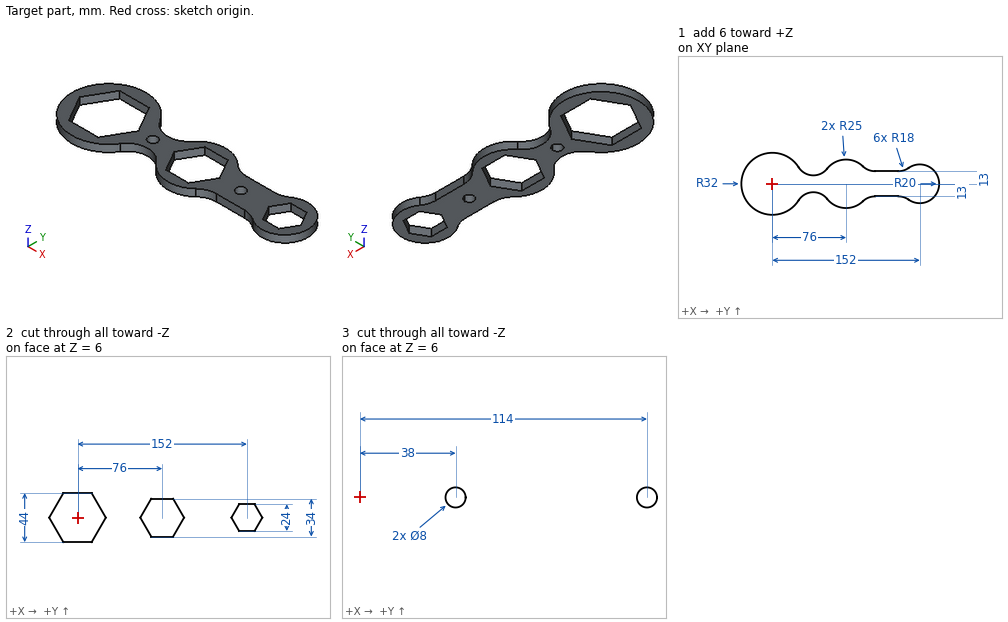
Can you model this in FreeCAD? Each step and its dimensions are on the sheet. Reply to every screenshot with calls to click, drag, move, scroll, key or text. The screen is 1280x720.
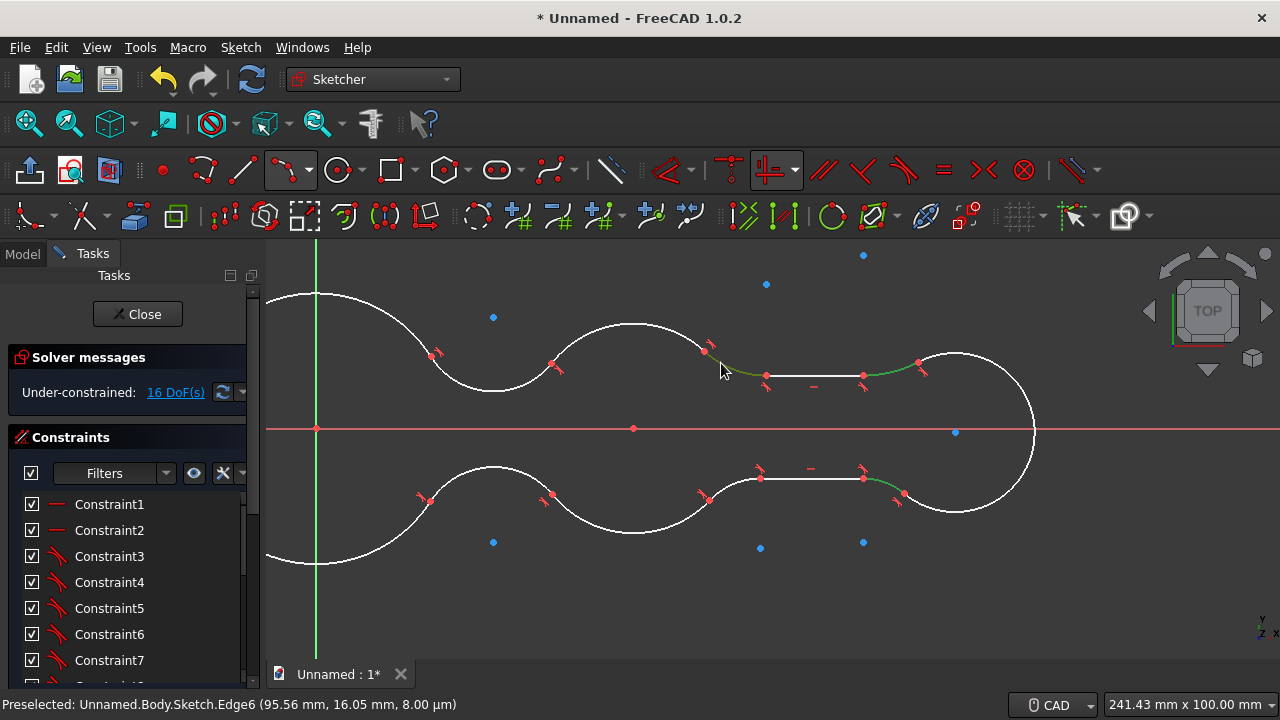
click(462, 385)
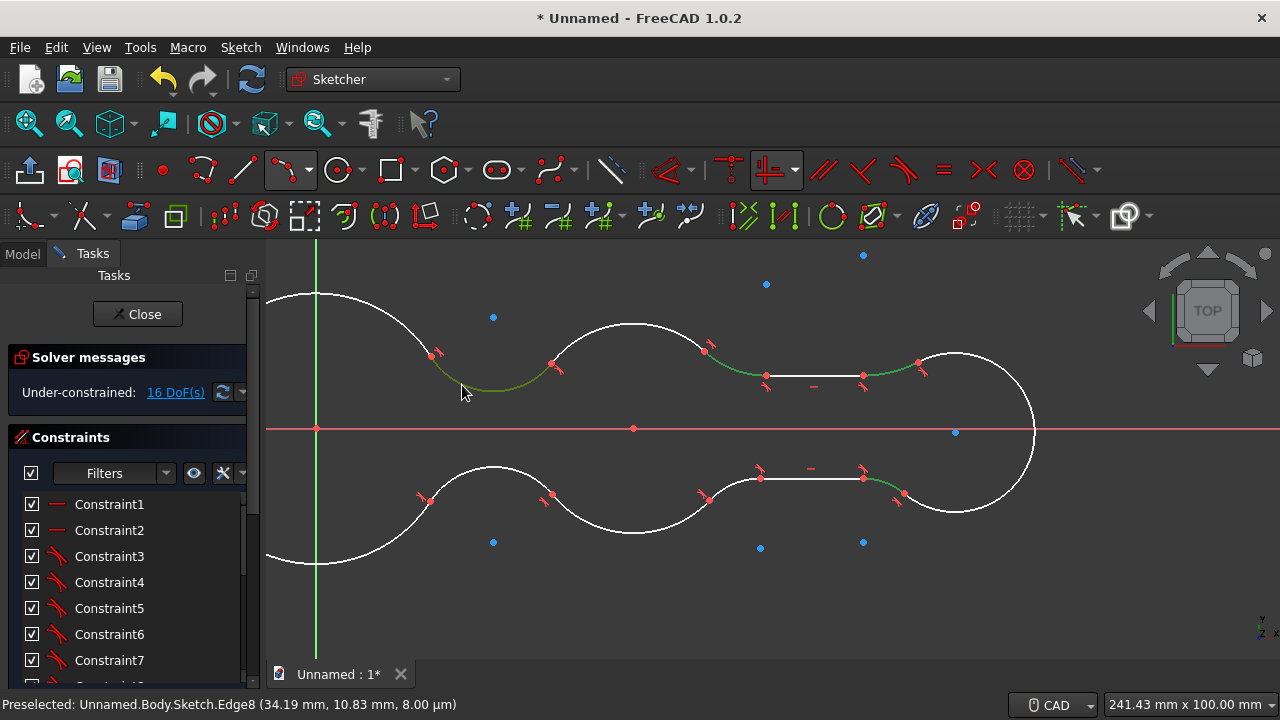
click(518, 471)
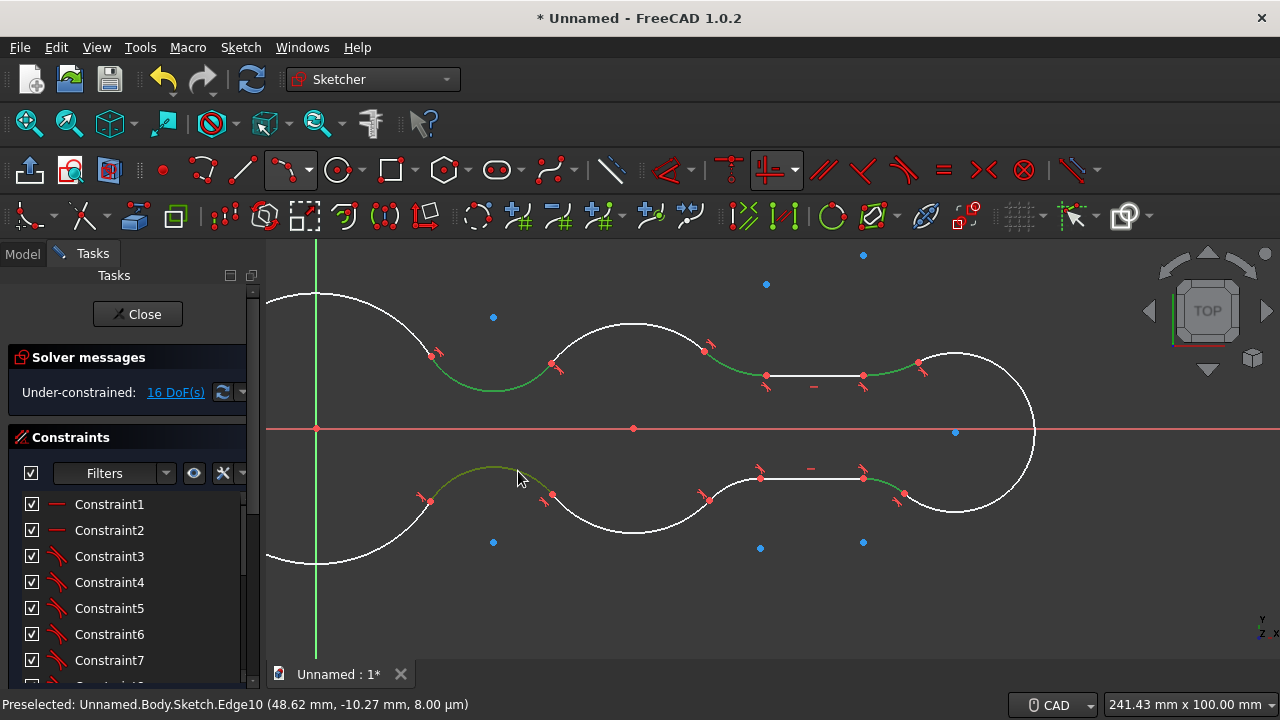
click(744, 481)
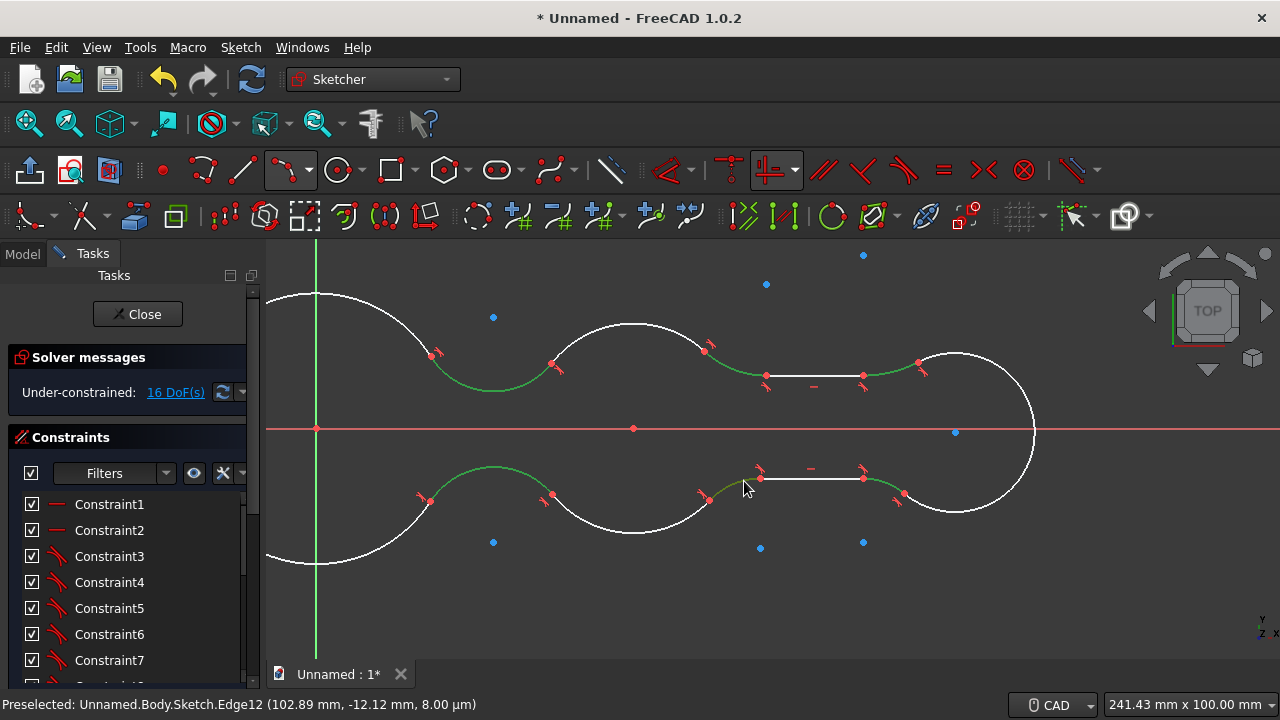
click(944, 170)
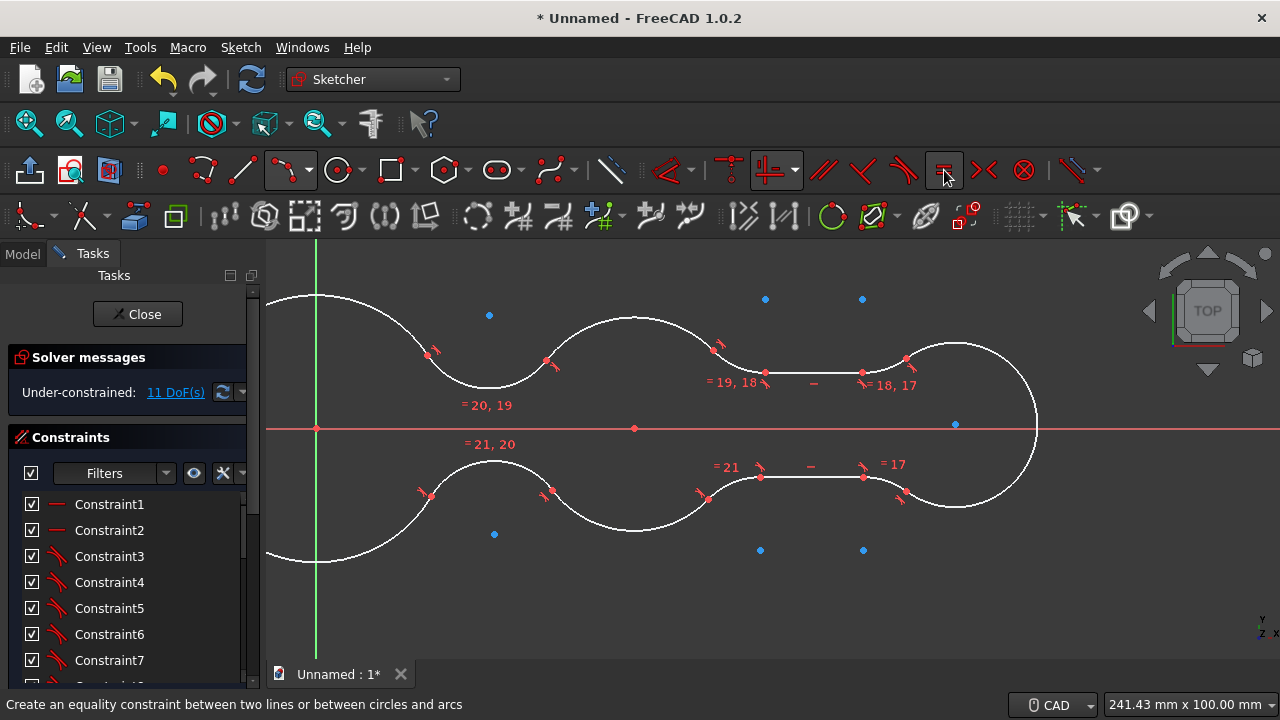
click(665, 322)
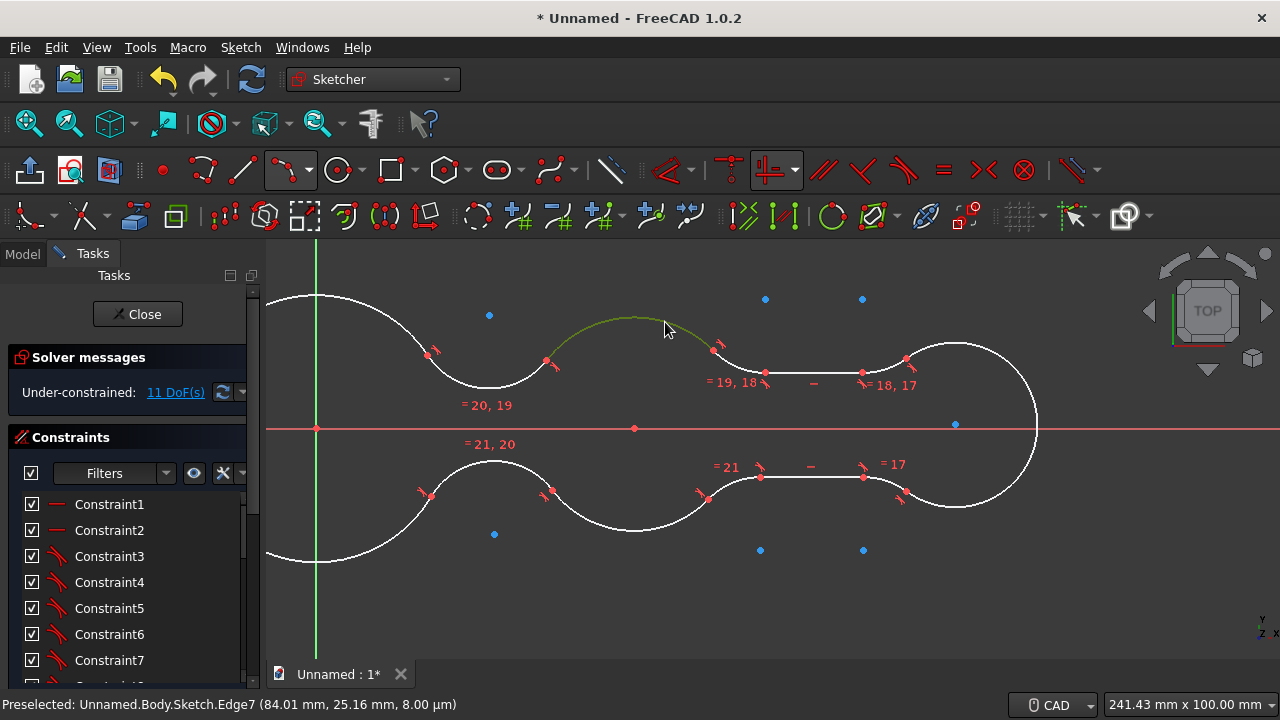
click(594, 523)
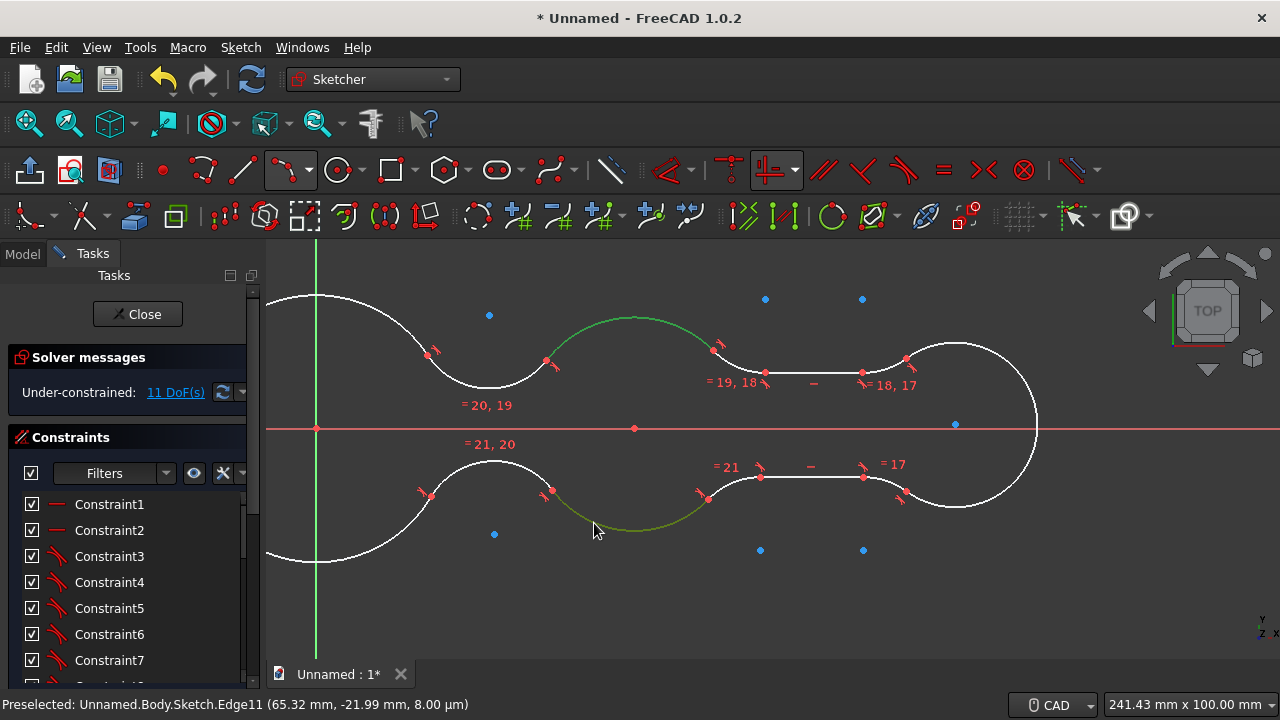
click(944, 170)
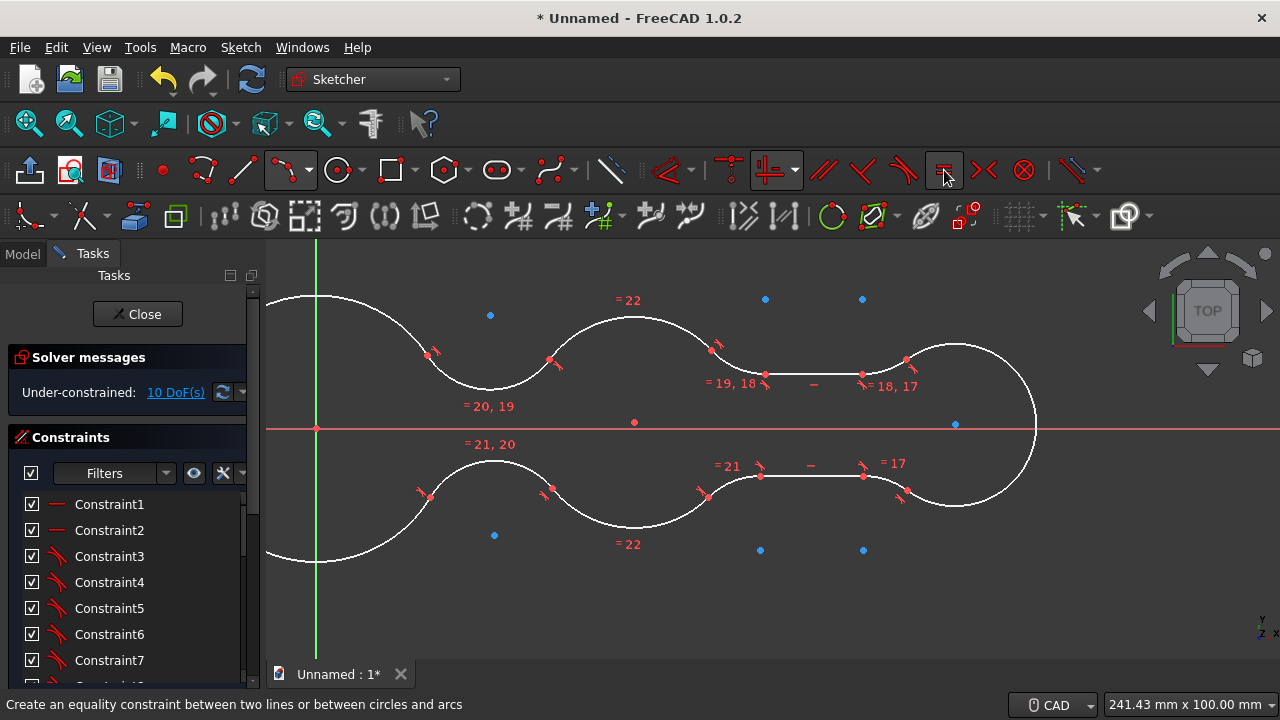
click(955, 425)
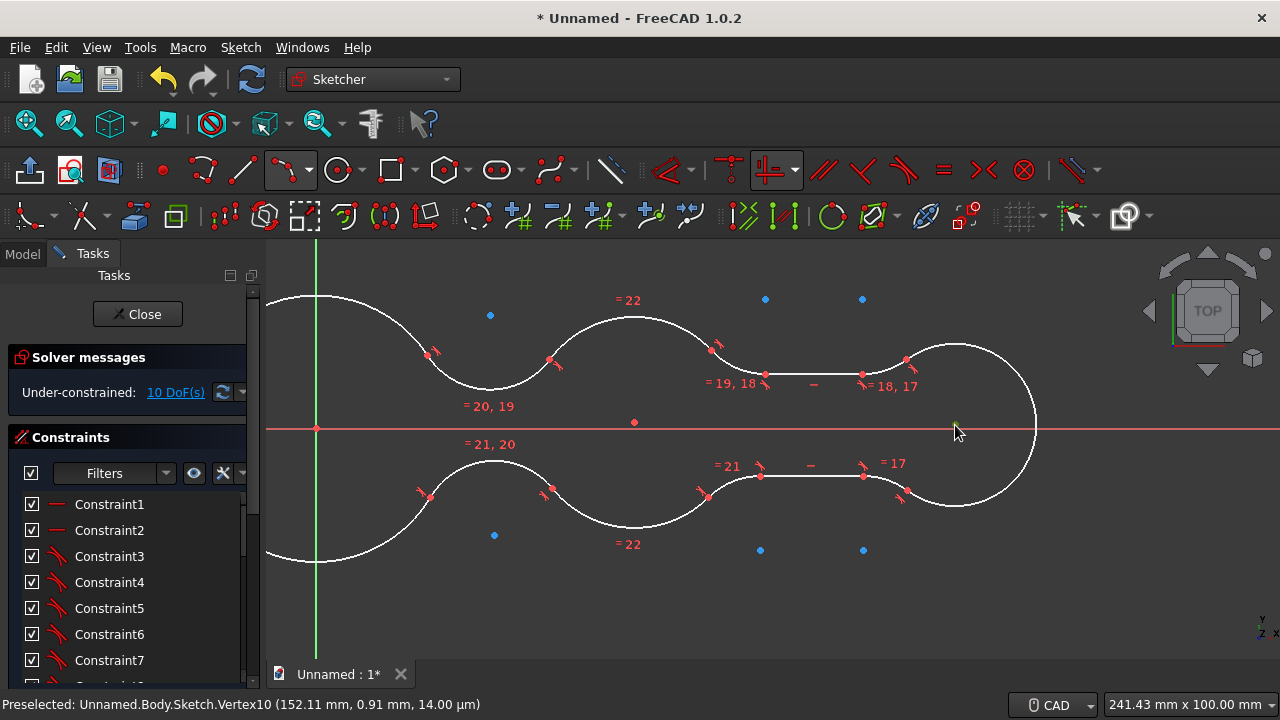
click(353, 429)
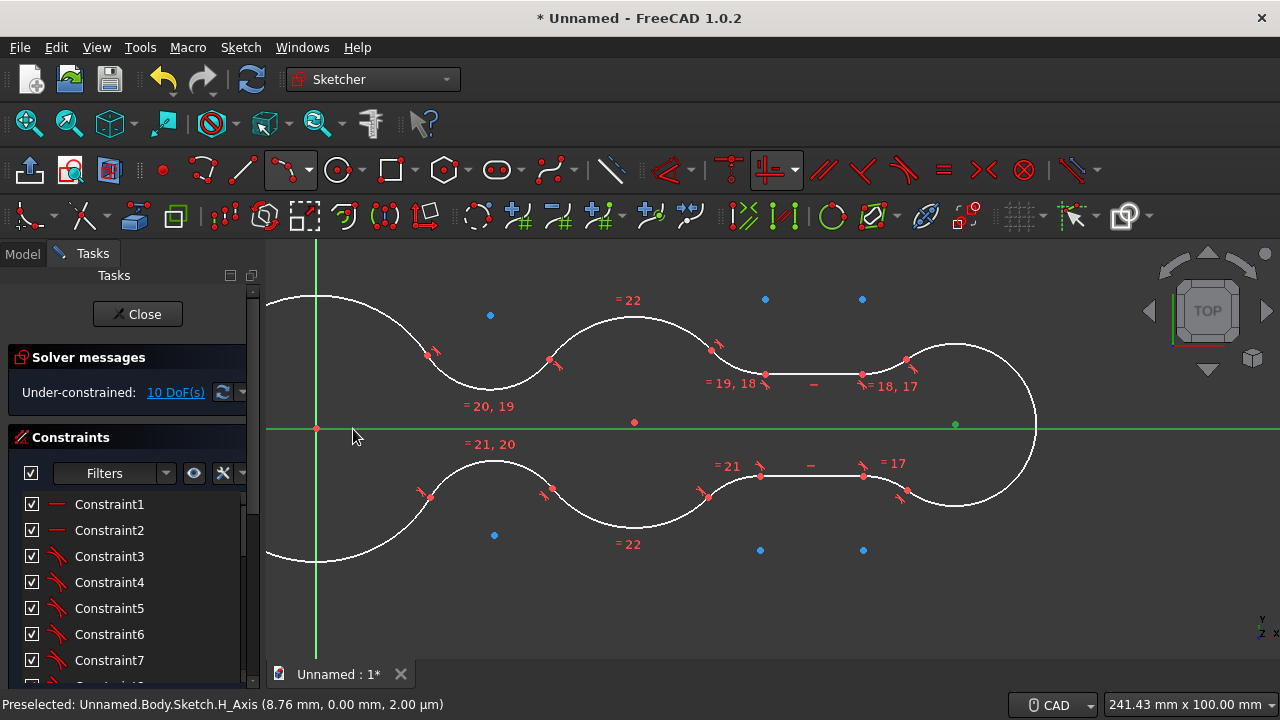
click(730, 170)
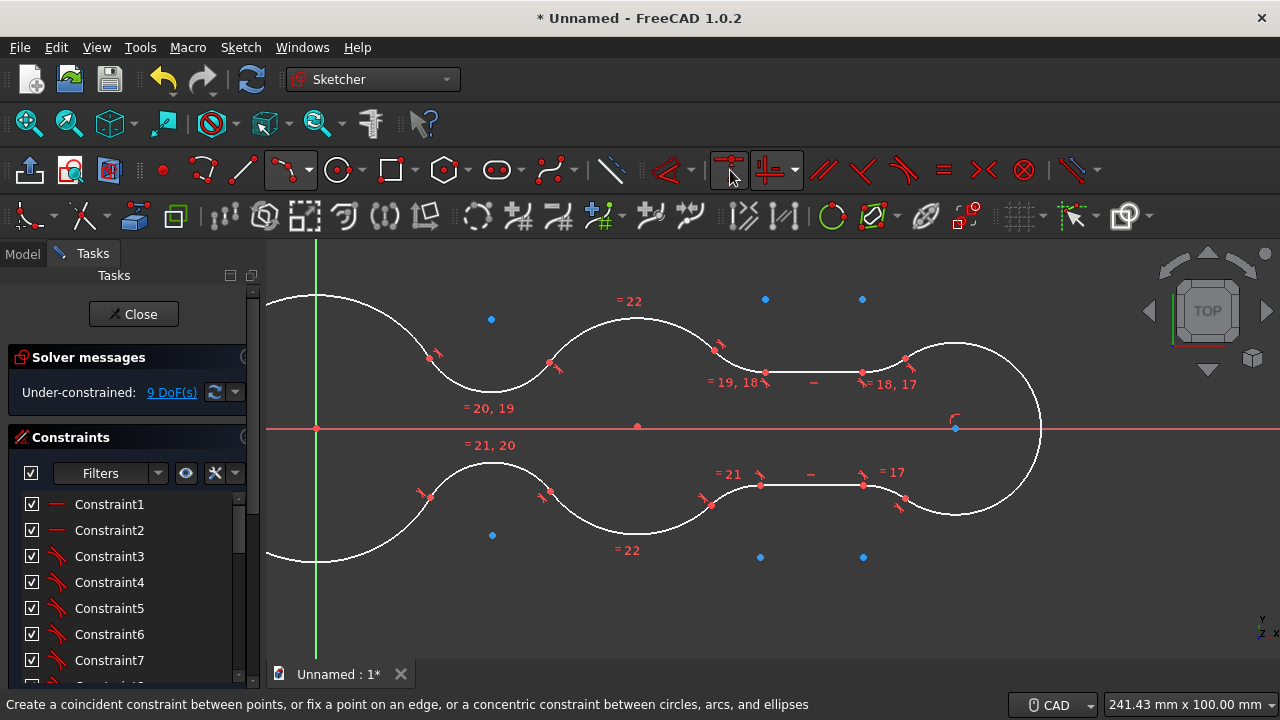
click(637, 426)